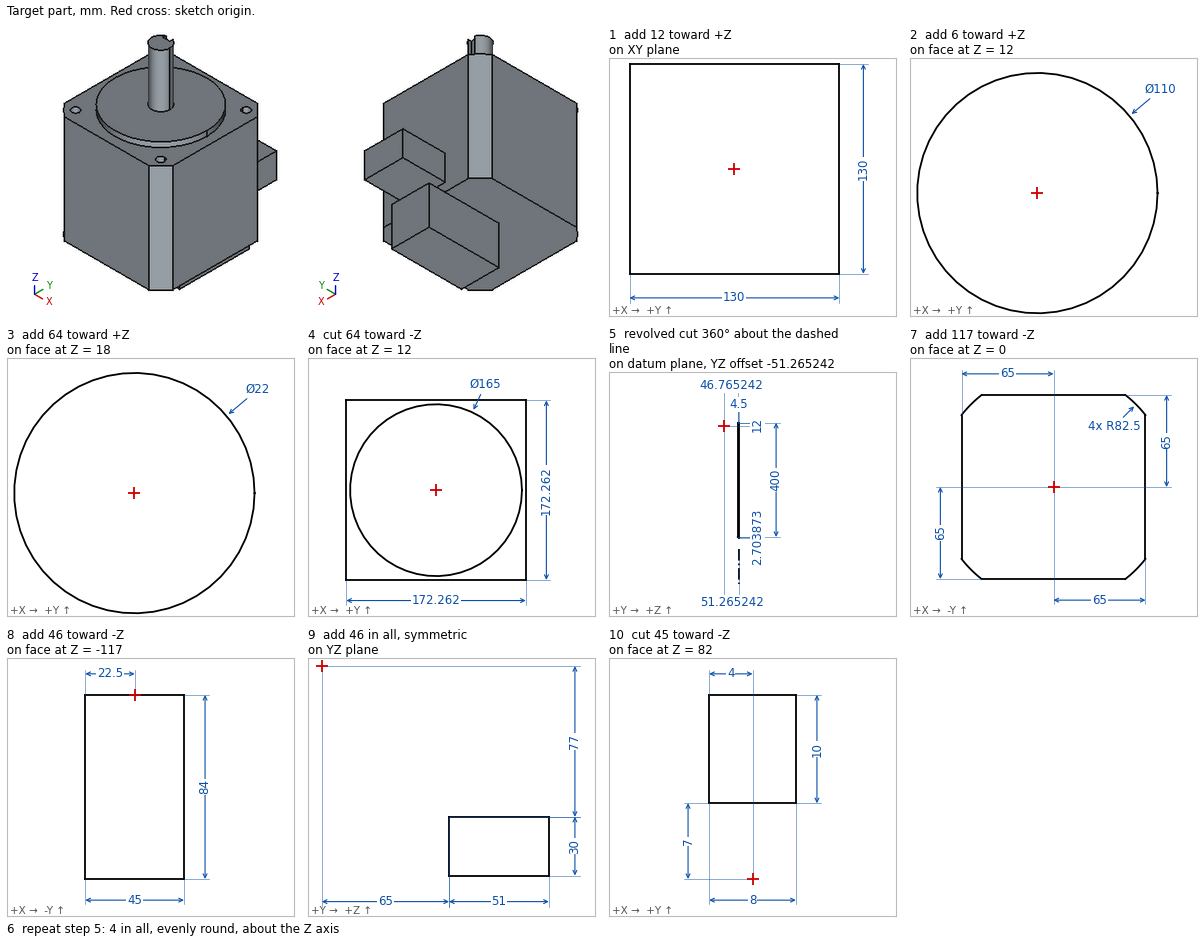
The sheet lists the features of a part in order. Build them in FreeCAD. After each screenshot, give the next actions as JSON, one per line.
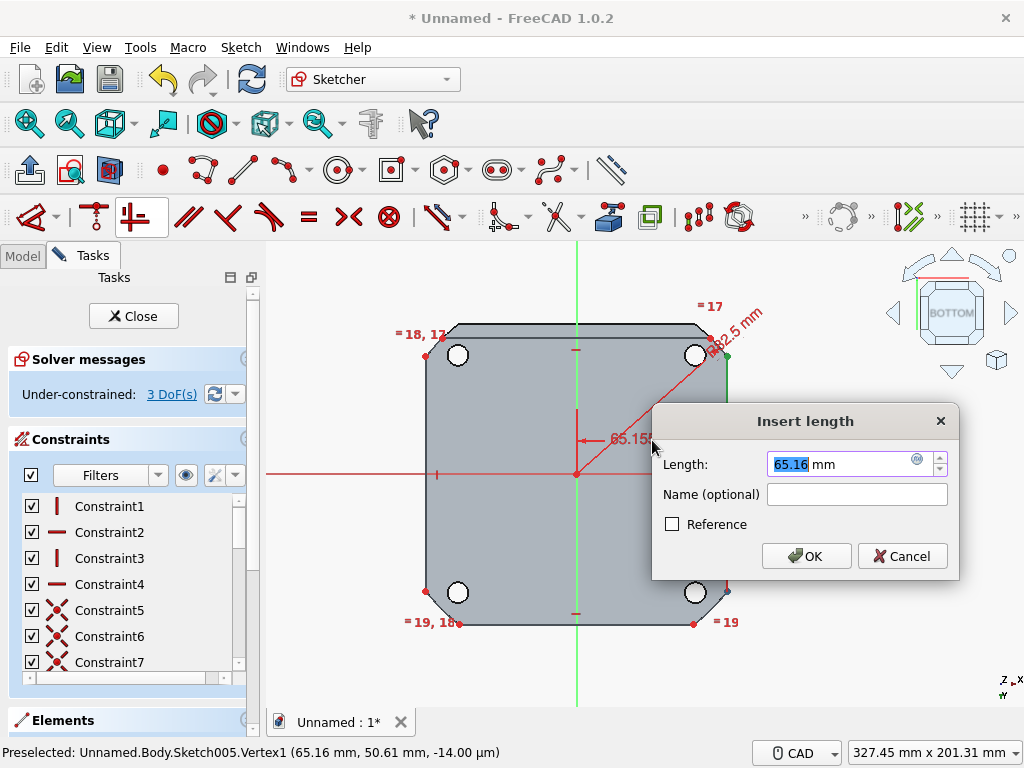
{"action": "type", "text": "65"}
{"action": "key", "text": "Return"}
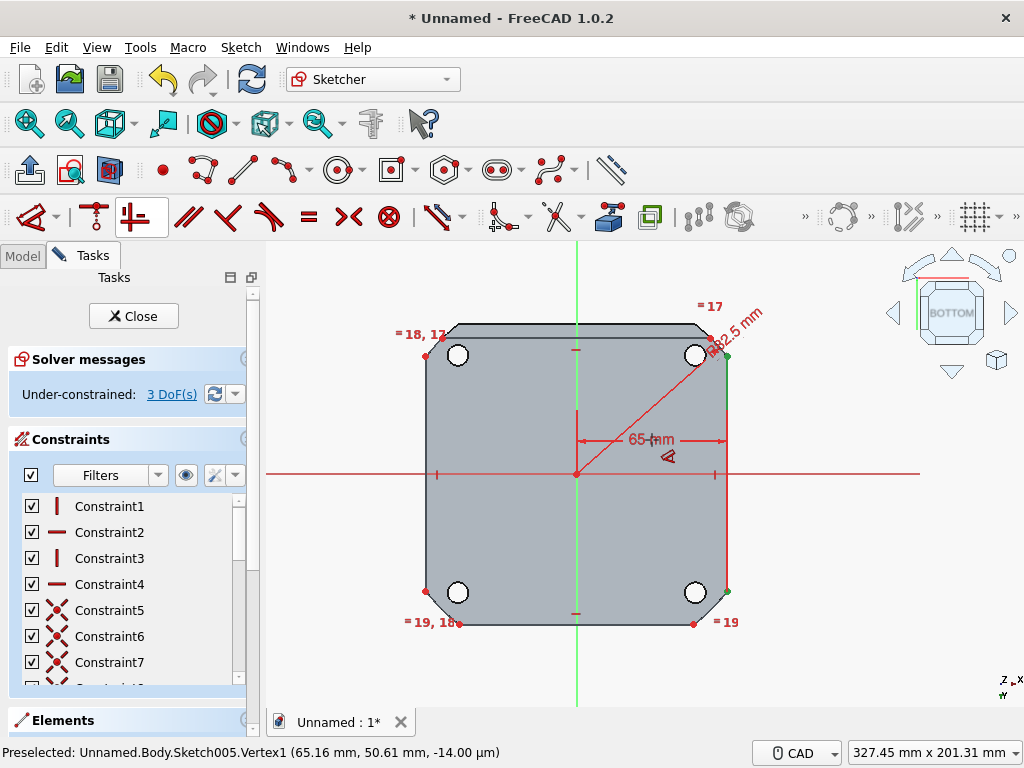
{"action": "left_click", "coordinate": [711, 338]}
{"action": "left_click", "coordinate": [745, 406]}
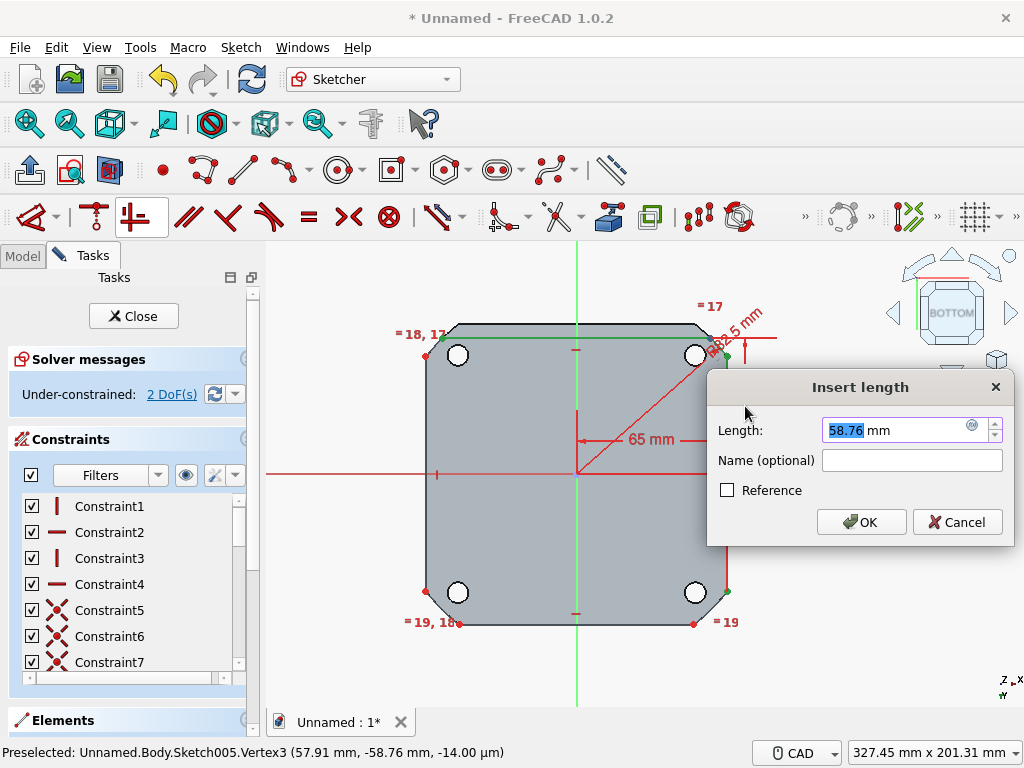
{"action": "type", "text": "65"}
{"action": "key", "text": "Return"}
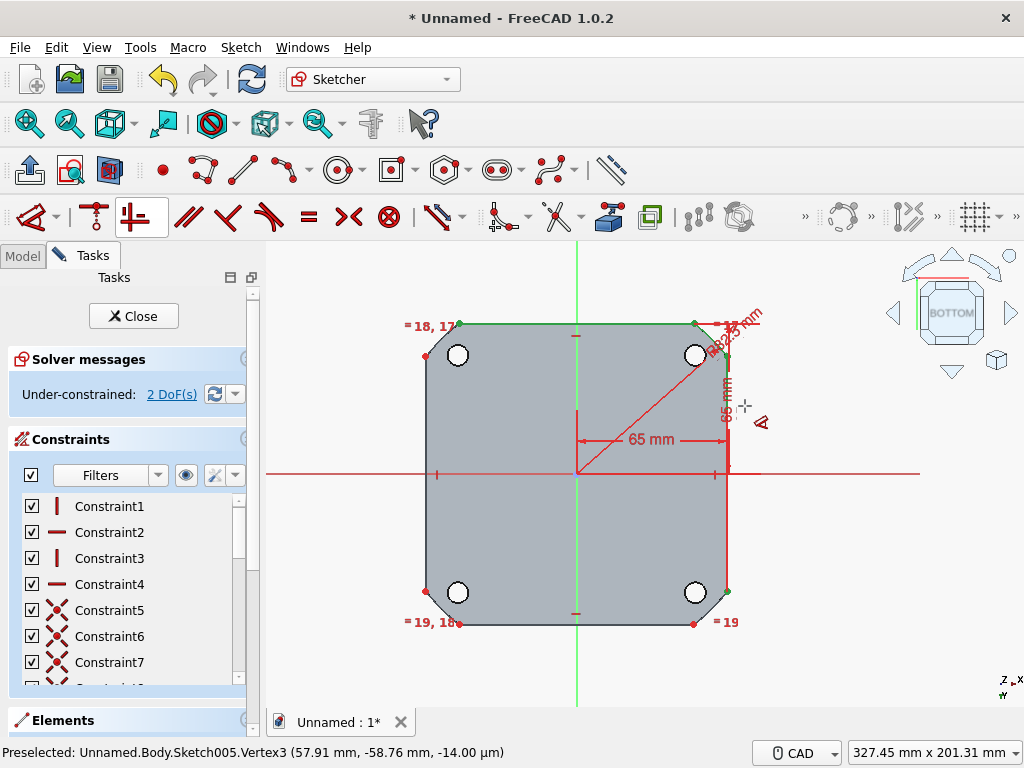
{"action": "left_click", "coordinate": [426, 357]}
{"action": "left_click", "coordinate": [501, 508]}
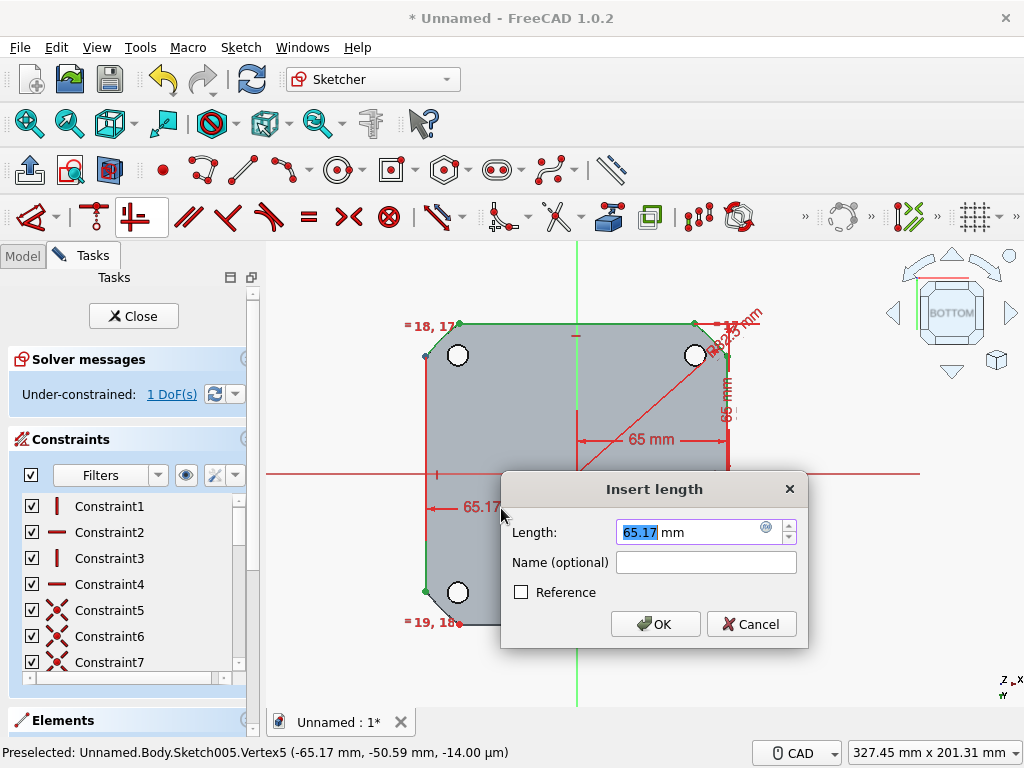
{"action": "type", "text": "65"}
{"action": "key", "text": "Return"}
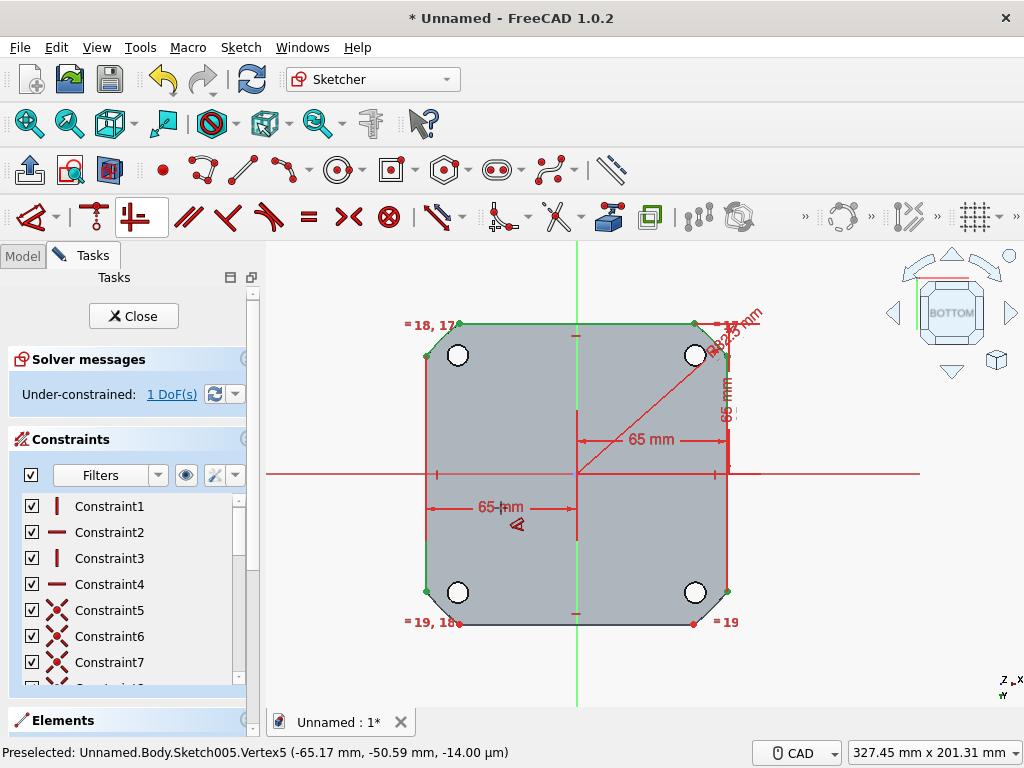
{"action": "left_click", "coordinate": [459, 625]}
{"action": "left_click", "coordinate": [611, 549]}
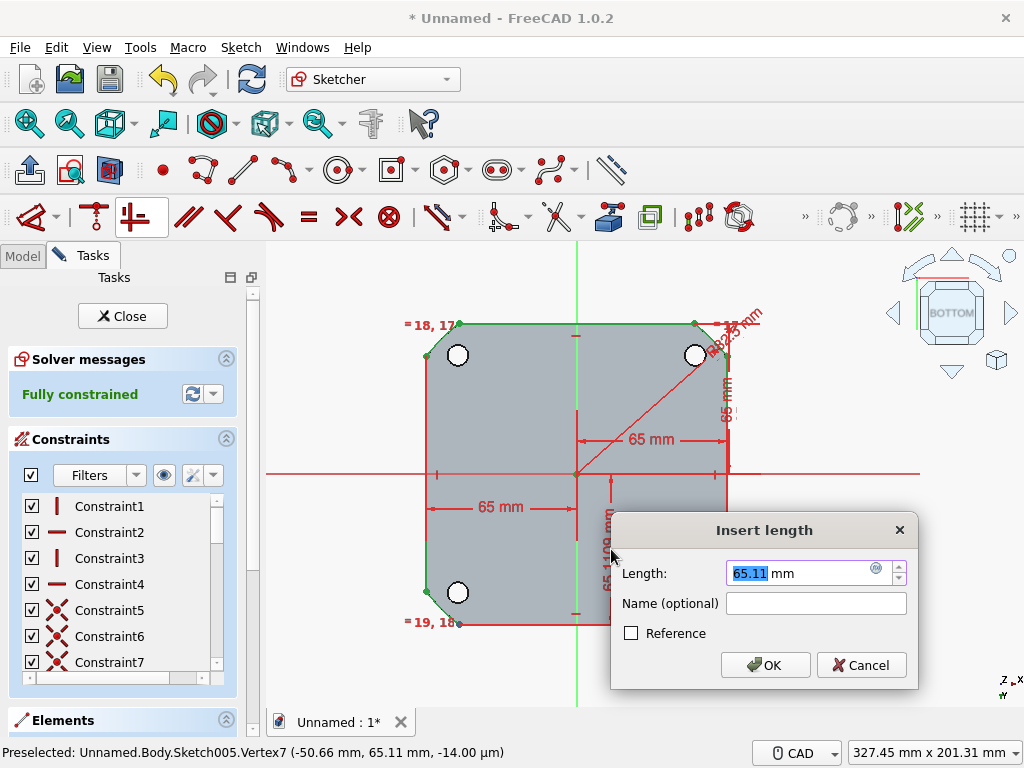
{"action": "type", "text": "65"}
{"action": "key", "text": "Return"}
{"action": "key", "text": "Escape"}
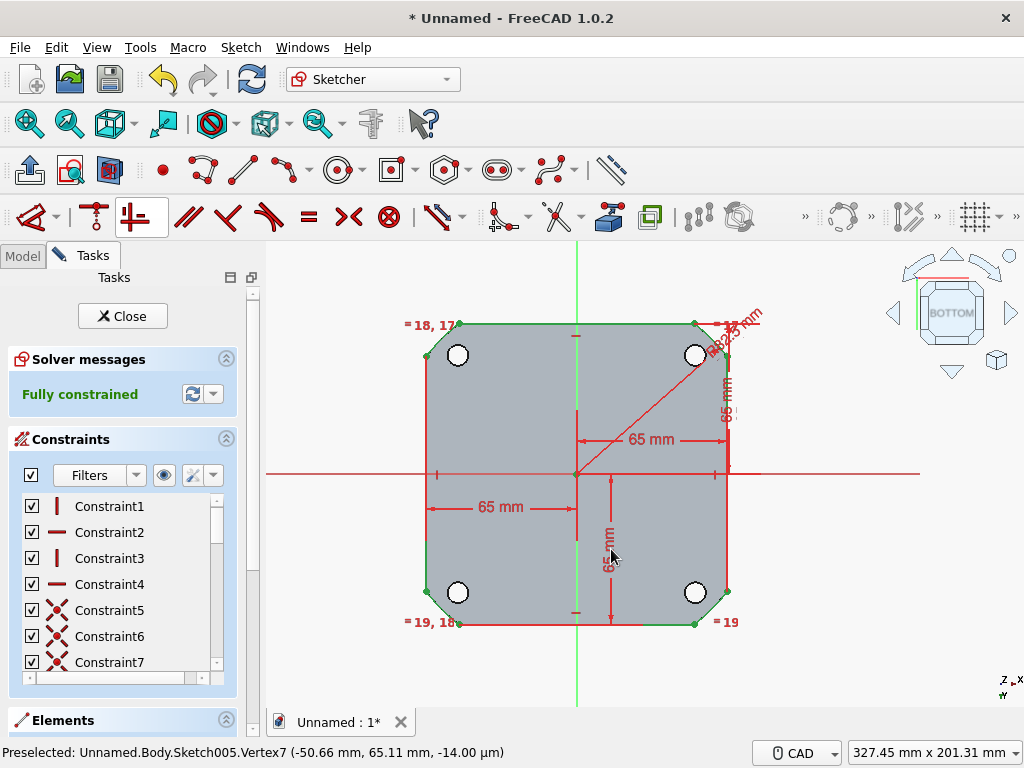
{"action": "left_click", "coordinate": [123, 316]}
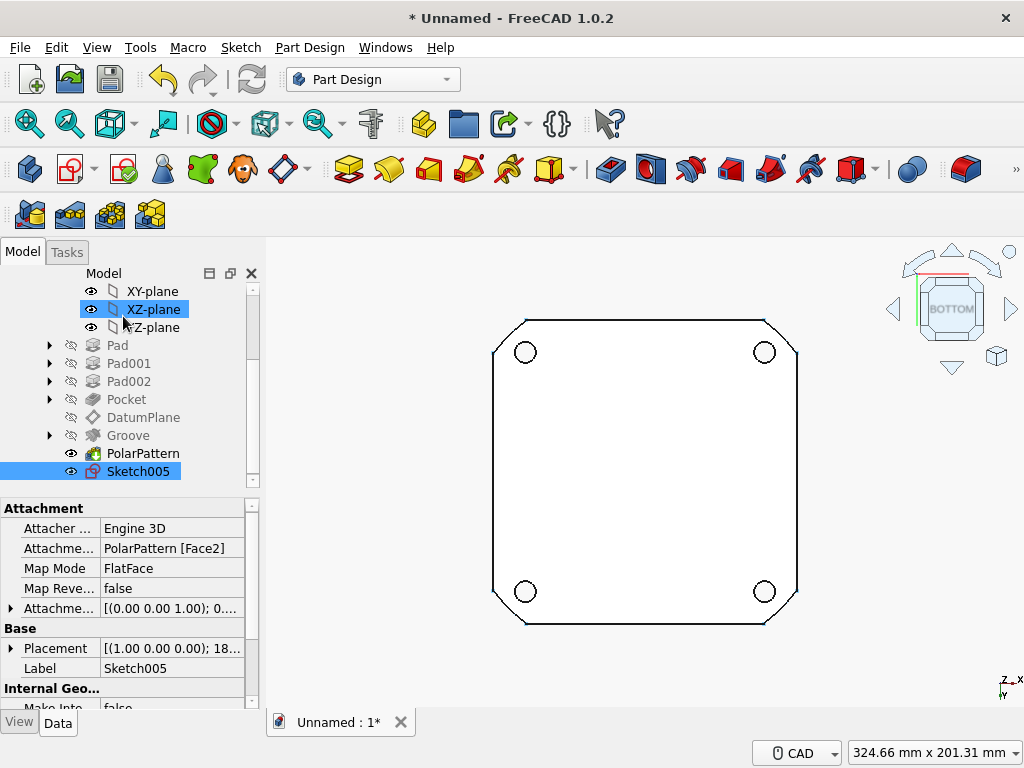
{"action": "left_click", "coordinate": [350, 170]}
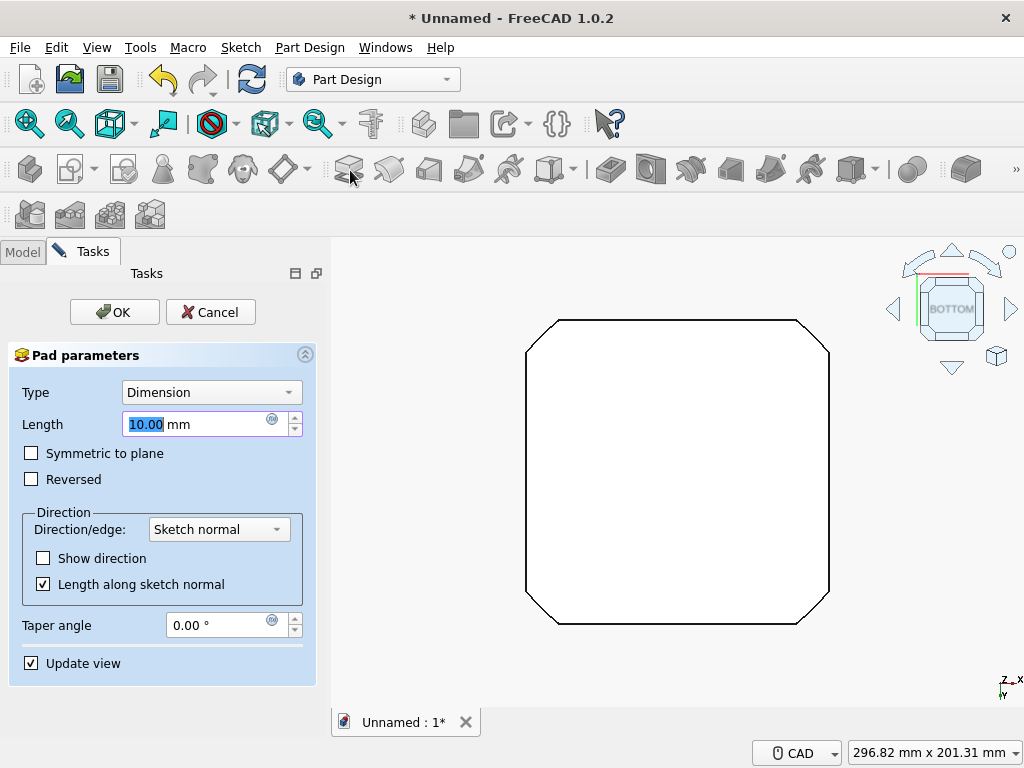
{"action": "type", "text": "117"}
{"action": "key", "text": "Tab"}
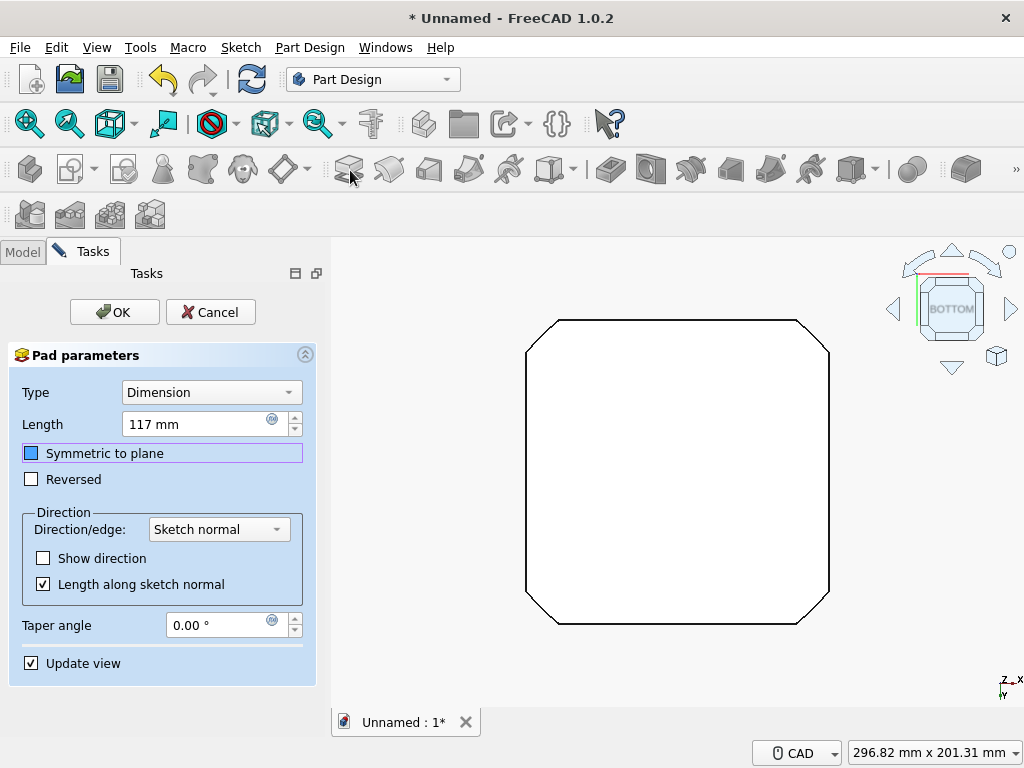
{"action": "left_click", "coordinate": [115, 312]}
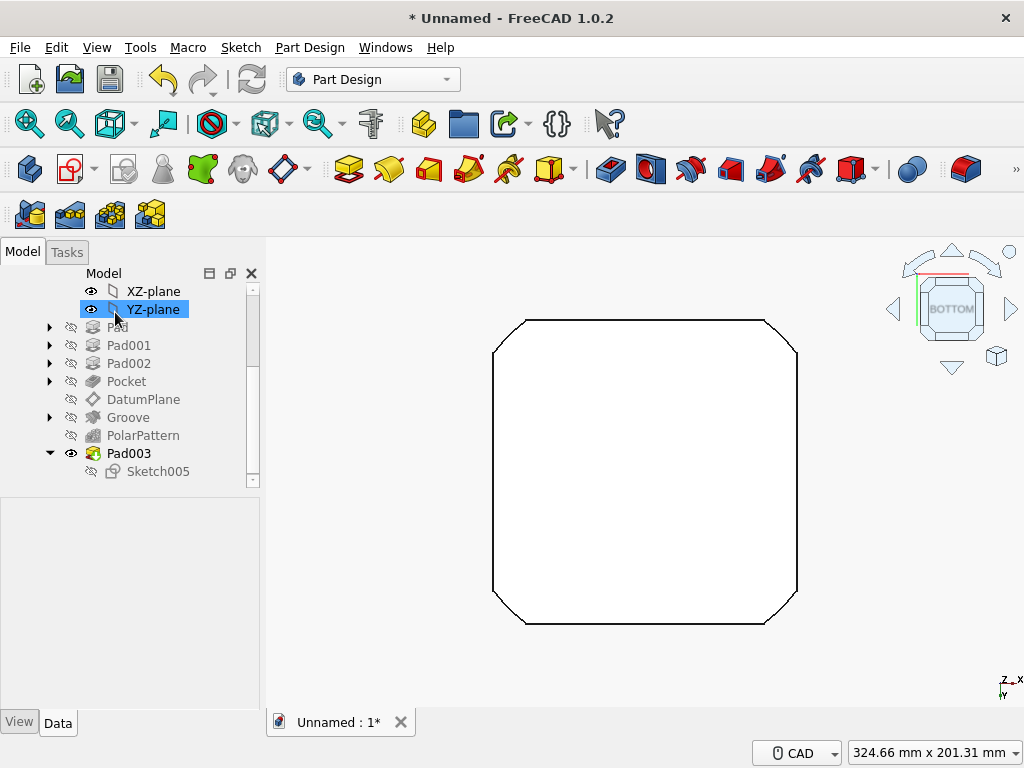
{"action": "left_click", "coordinate": [645, 471]}